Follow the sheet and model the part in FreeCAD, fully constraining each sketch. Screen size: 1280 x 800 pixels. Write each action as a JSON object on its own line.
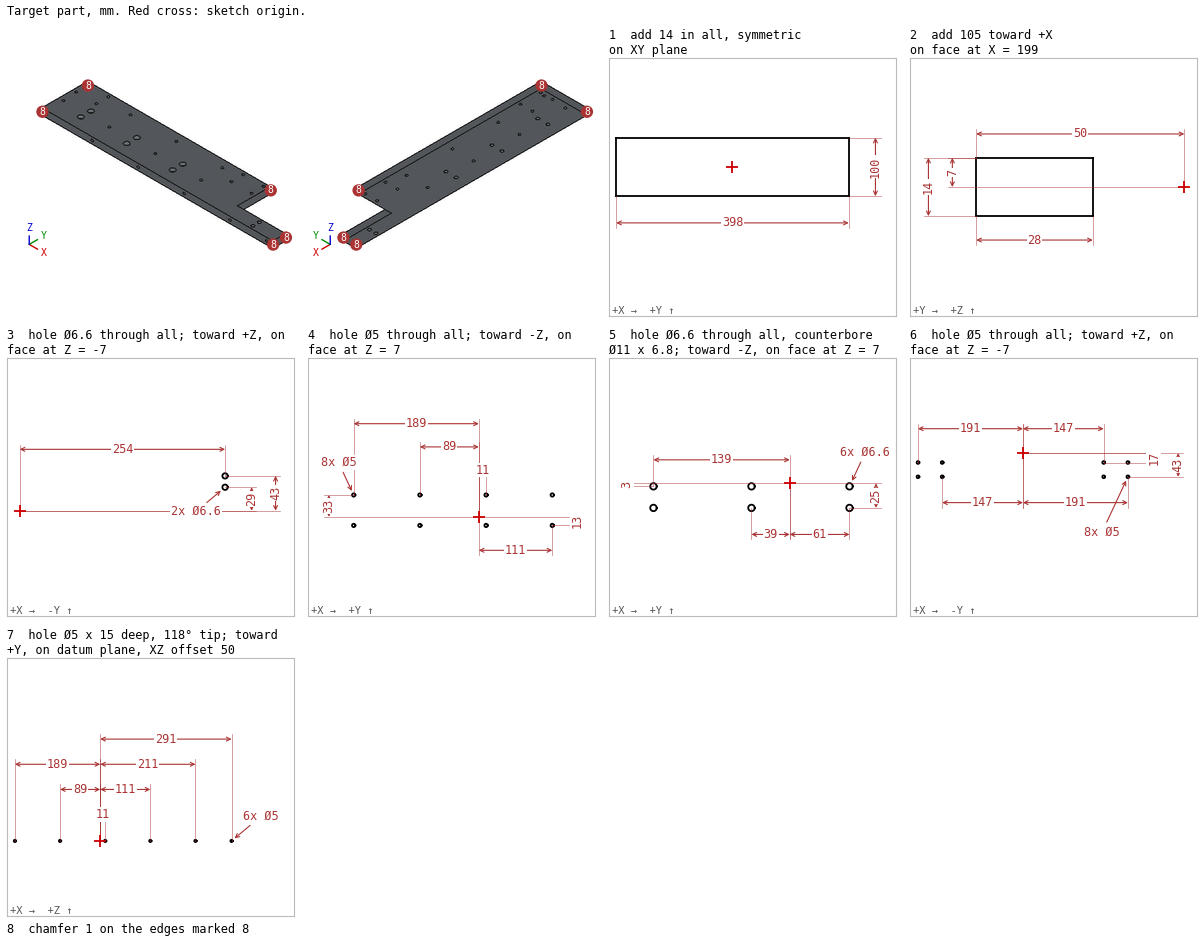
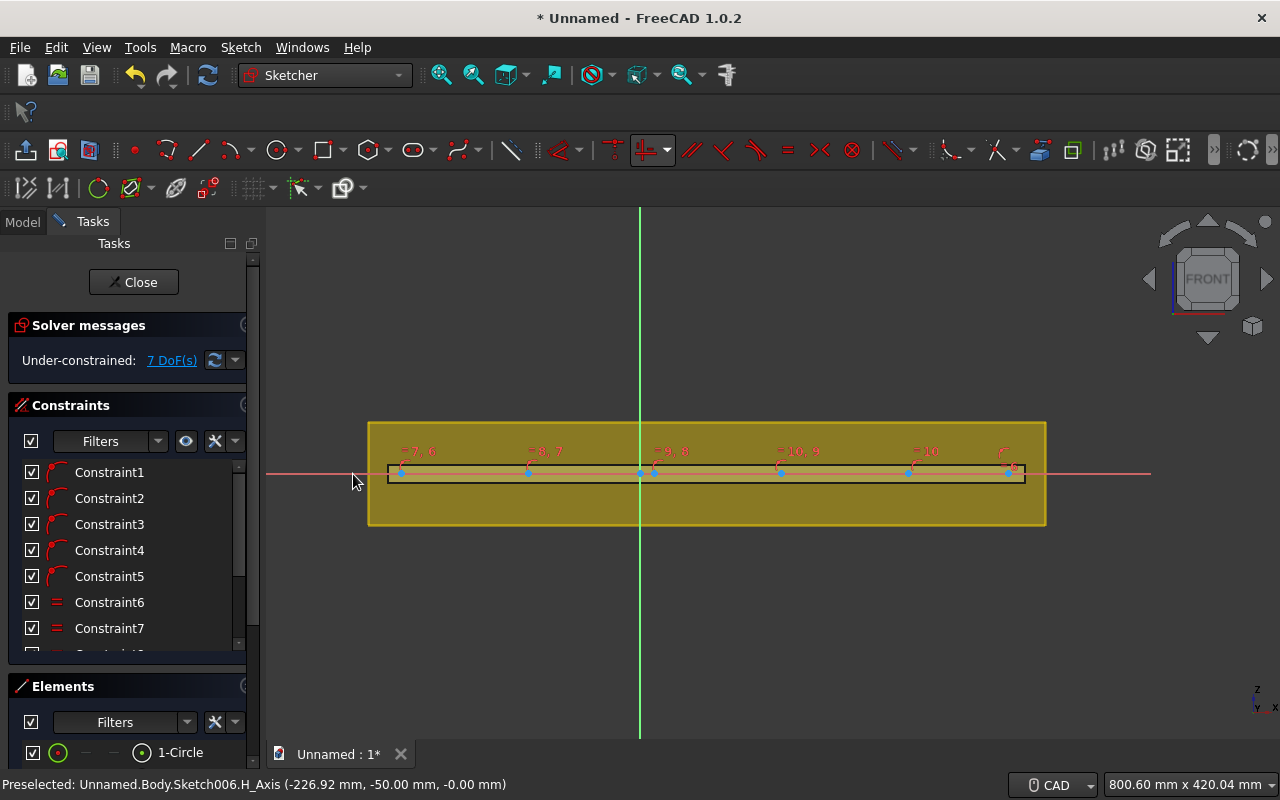
{"action": "key", "text": "d"}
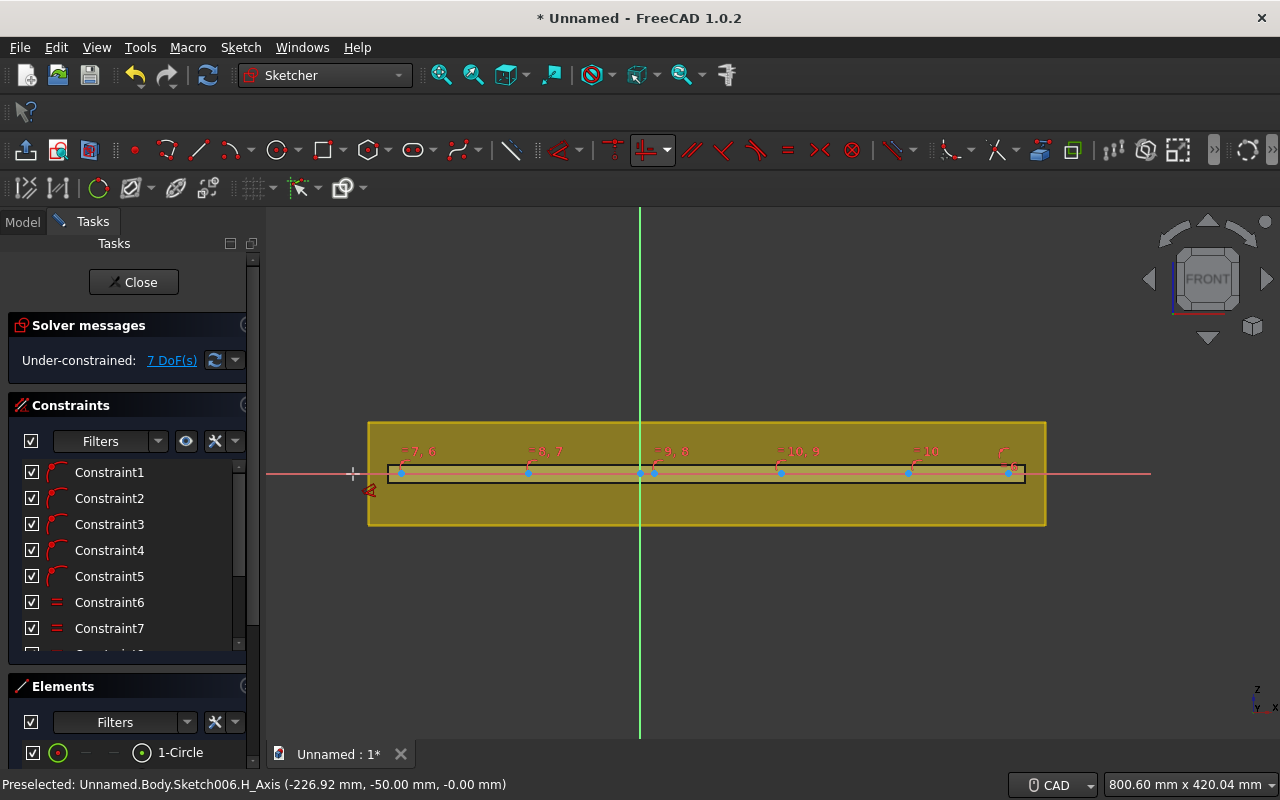
{"action": "scroll", "coordinate": [1009, 472], "scroll_direction": "up", "scroll_amount": 10}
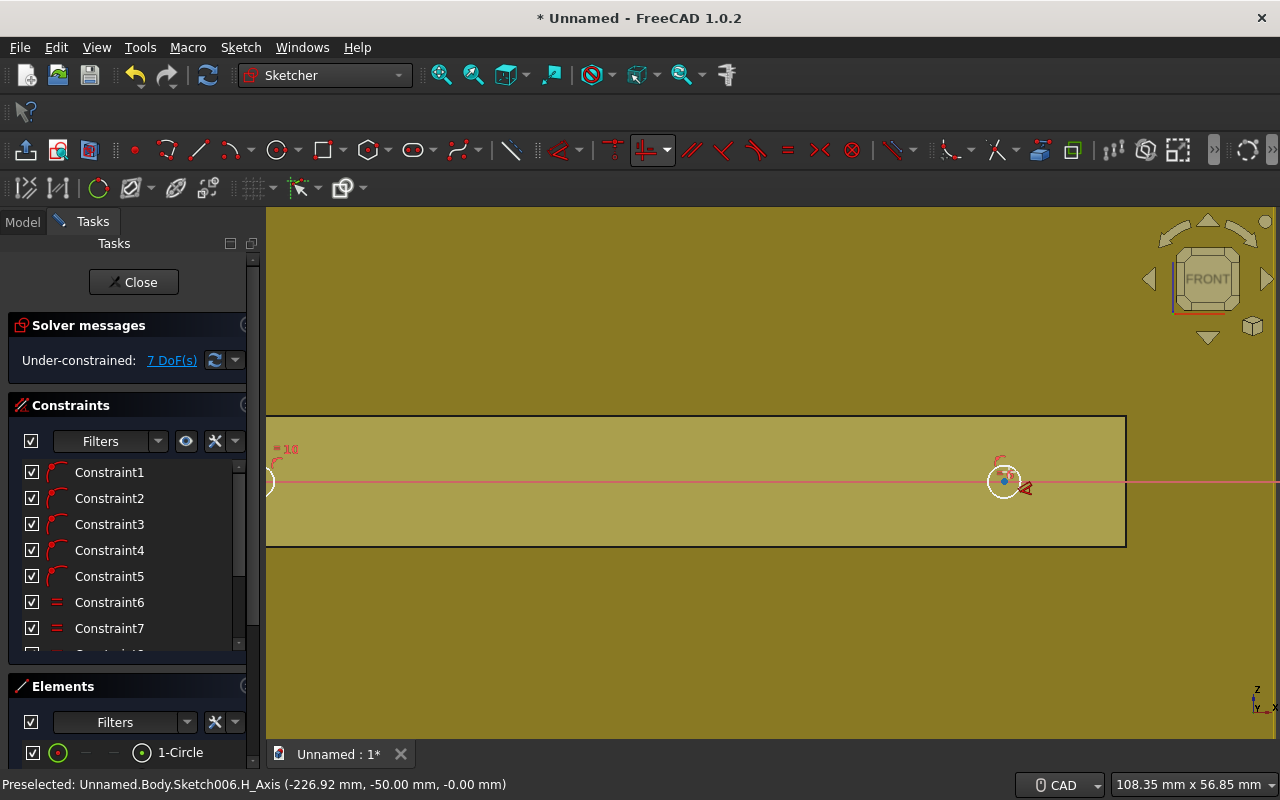
{"action": "left_click", "coordinate": [1005, 466]}
{"action": "left_click", "coordinate": [1006, 434]}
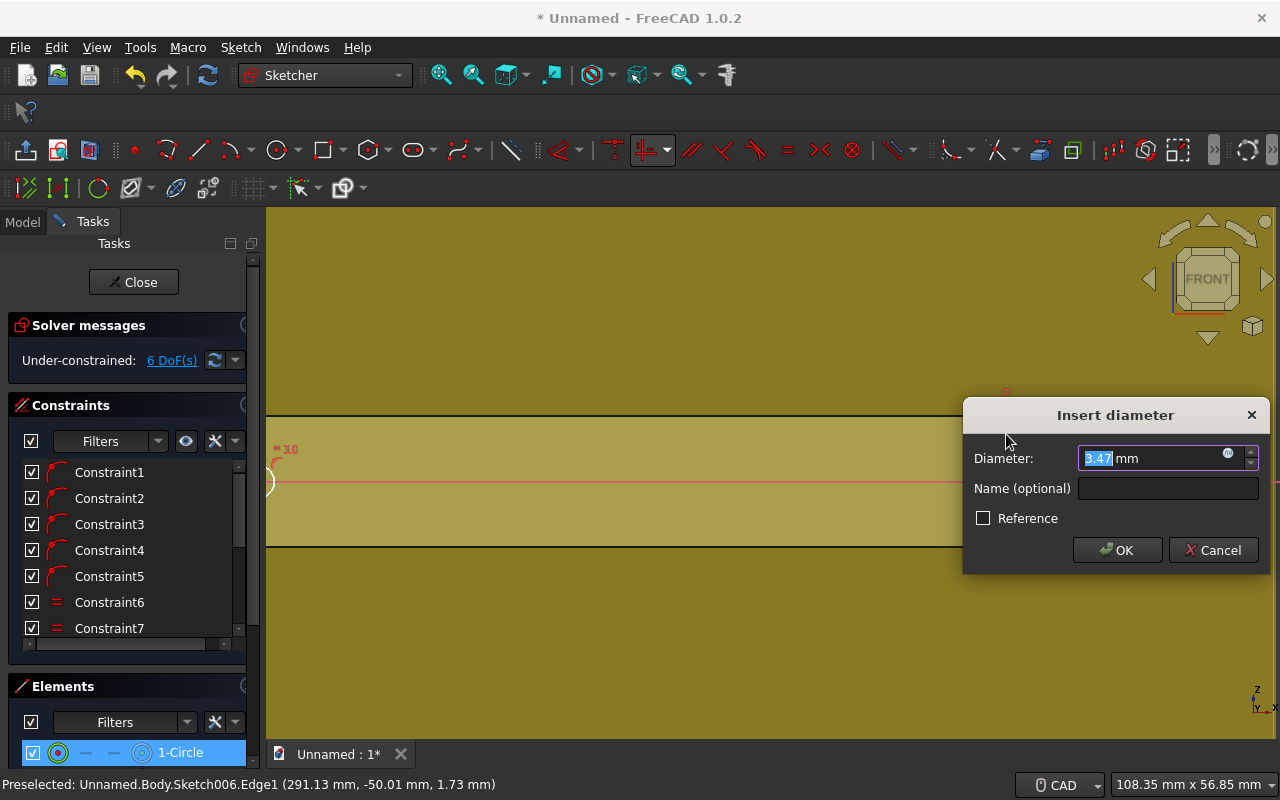
{"action": "type", "text": "5"}
{"action": "key", "text": "Return"}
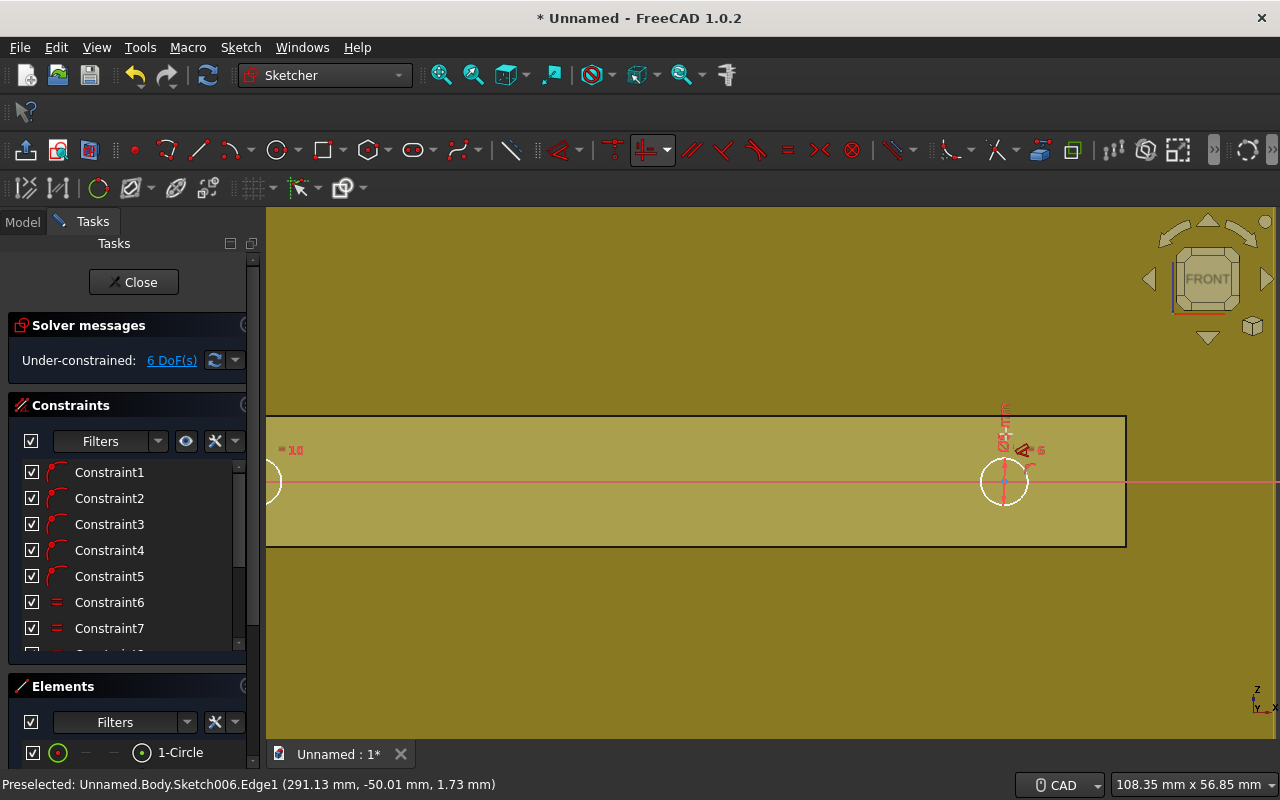
{"action": "scroll", "coordinate": [1009, 472], "scroll_direction": "down", "scroll_amount": 10}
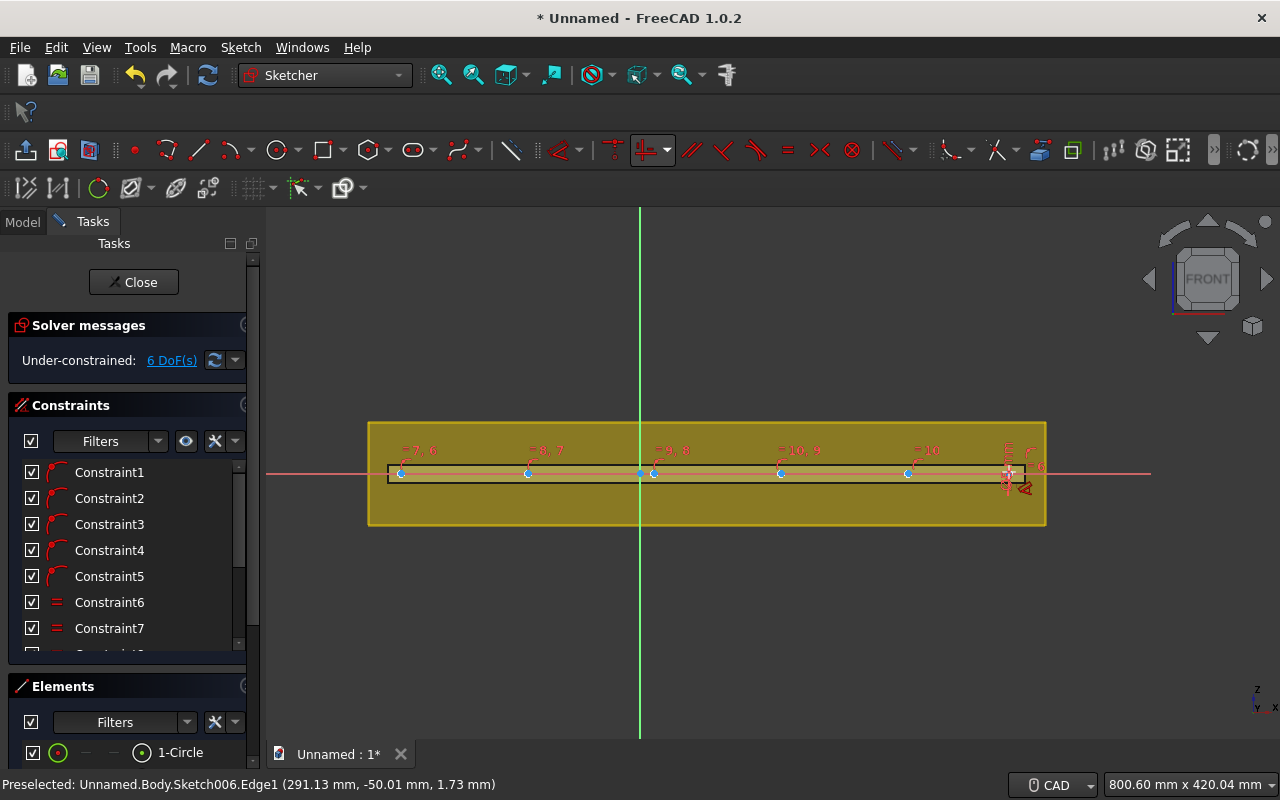
{"action": "left_click", "coordinate": [528, 474]}
{"action": "left_click", "coordinate": [584, 508]}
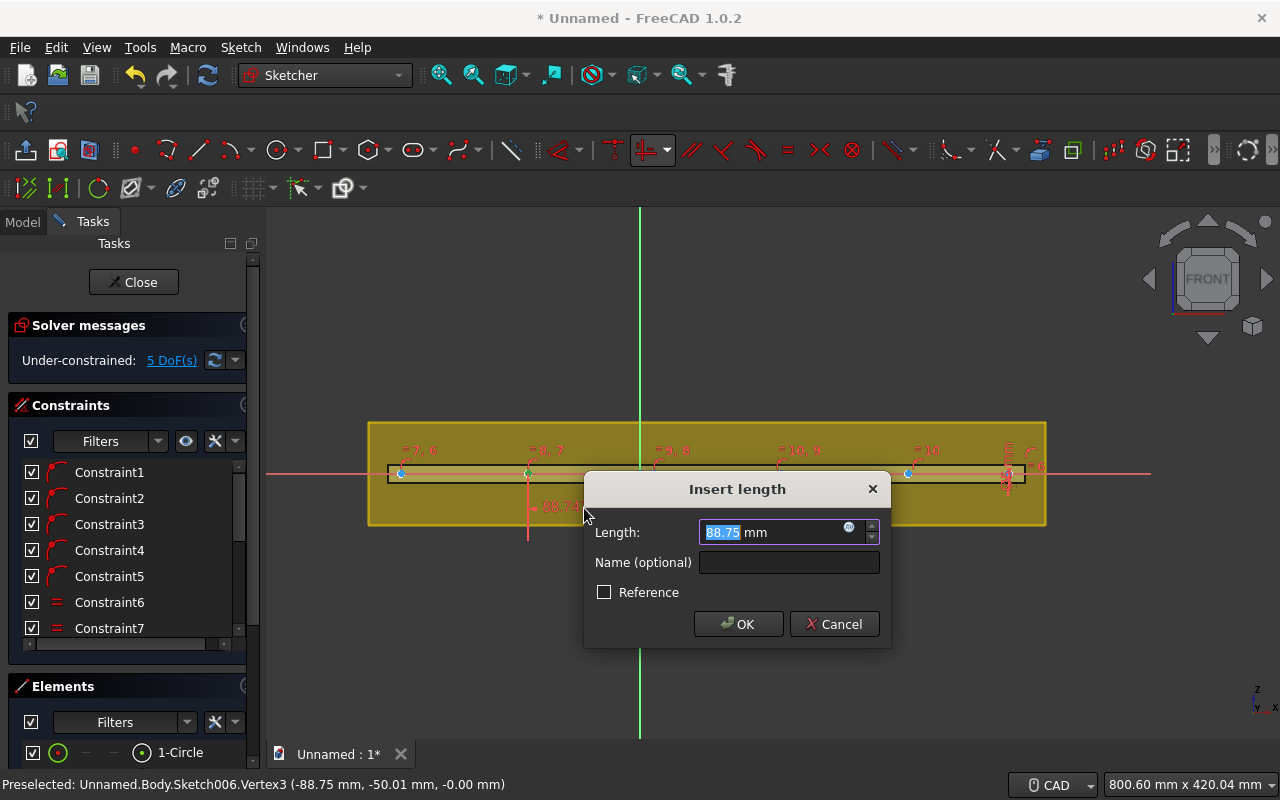
{"action": "type", "text": "89"}
{"action": "key", "text": "Return"}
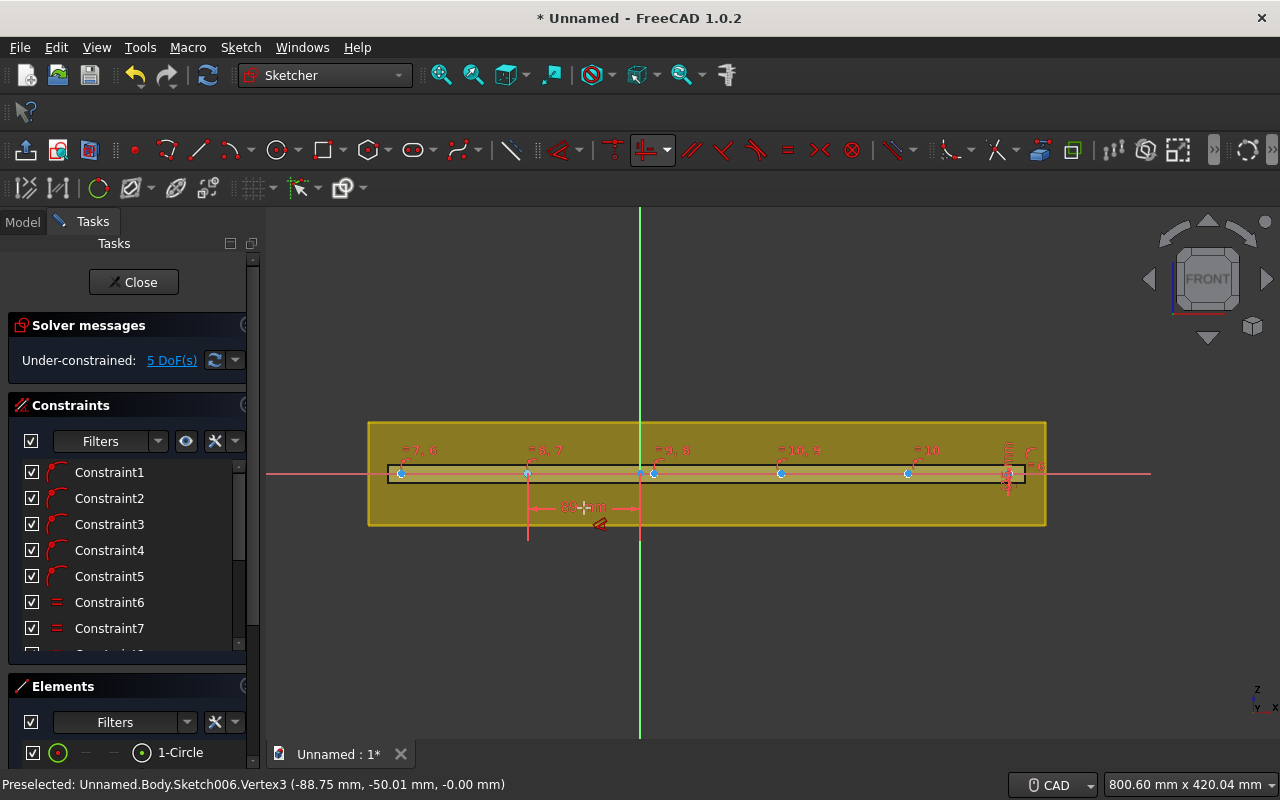
{"action": "scroll", "coordinate": [654, 474], "scroll_direction": "up", "scroll_amount": 6}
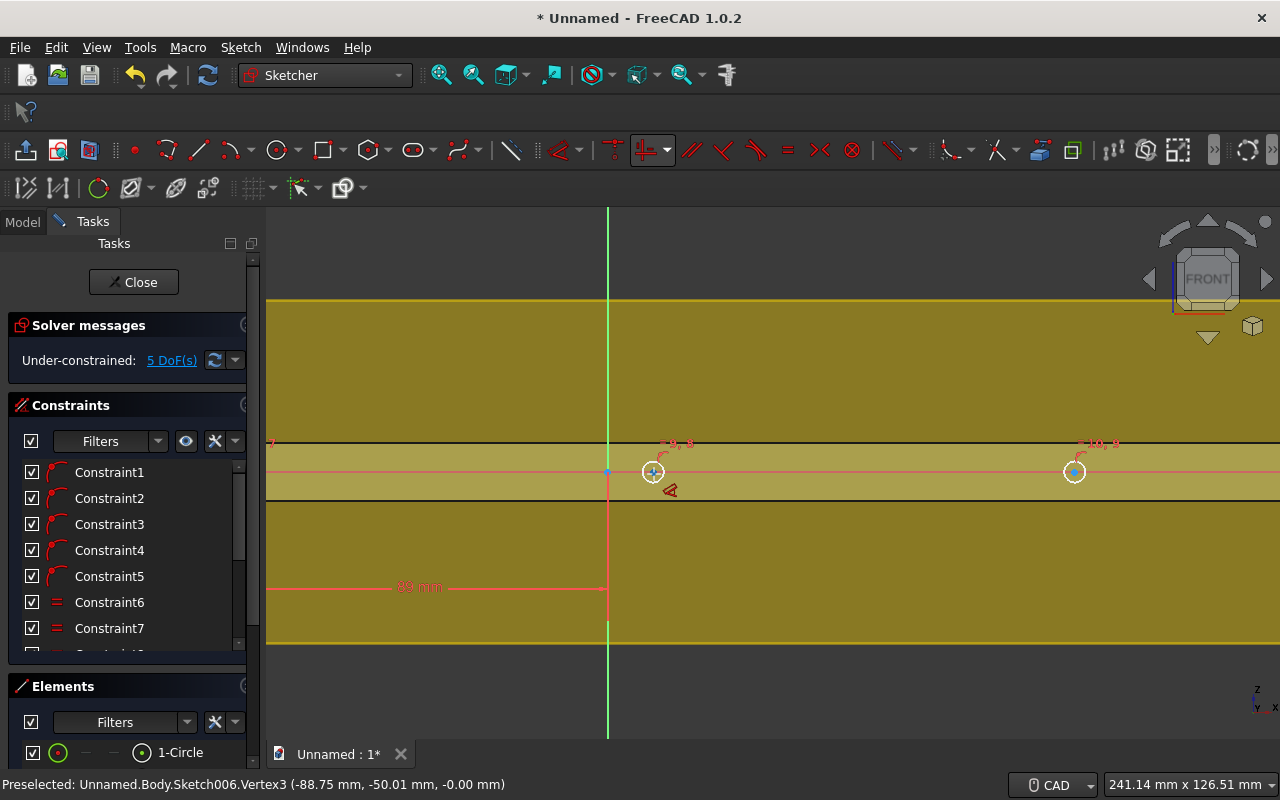
{"action": "left_click", "coordinate": [653, 472]}
{"action": "left_click", "coordinate": [631, 506]}